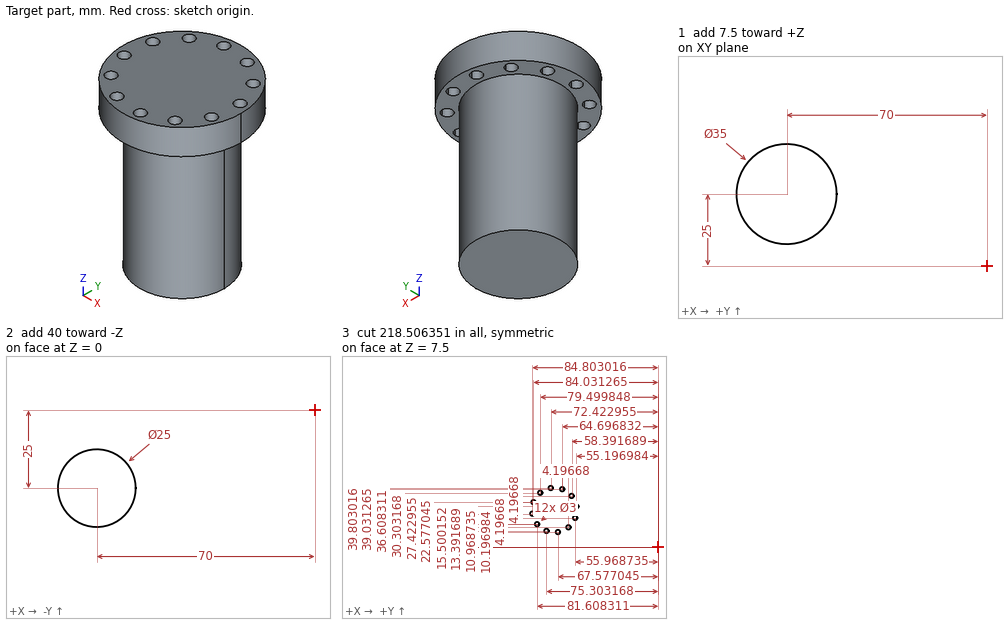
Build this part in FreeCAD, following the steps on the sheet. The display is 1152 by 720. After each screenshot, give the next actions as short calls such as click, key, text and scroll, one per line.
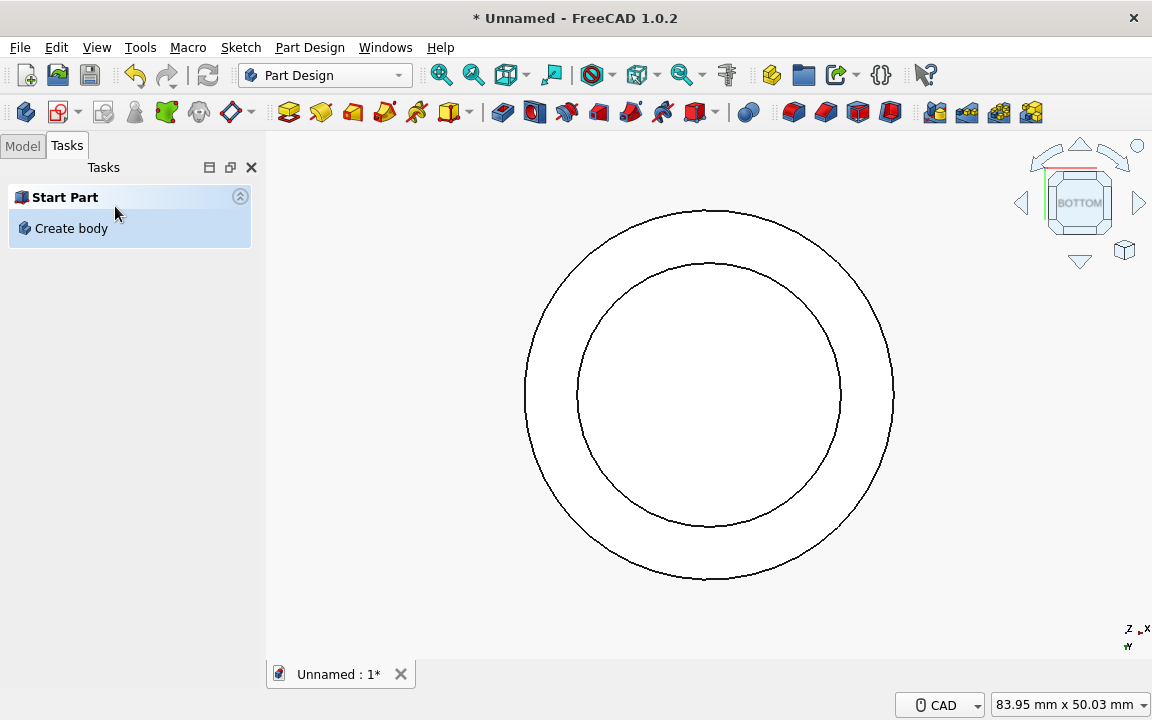
key(0)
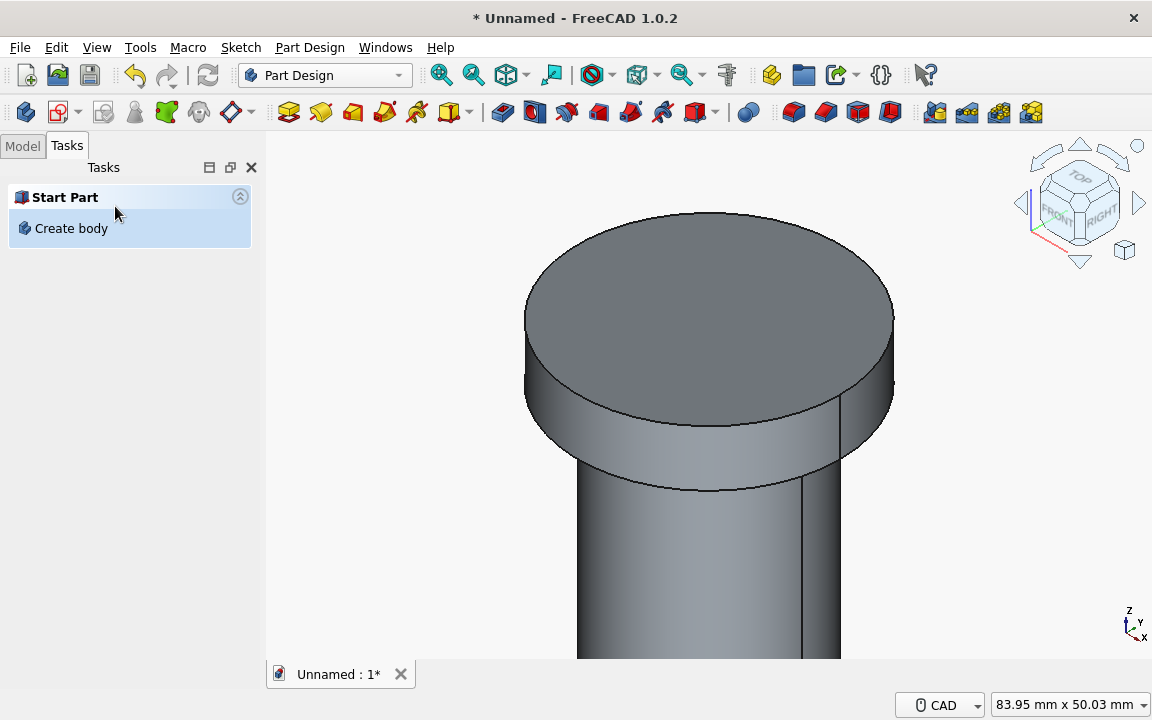
click(442, 76)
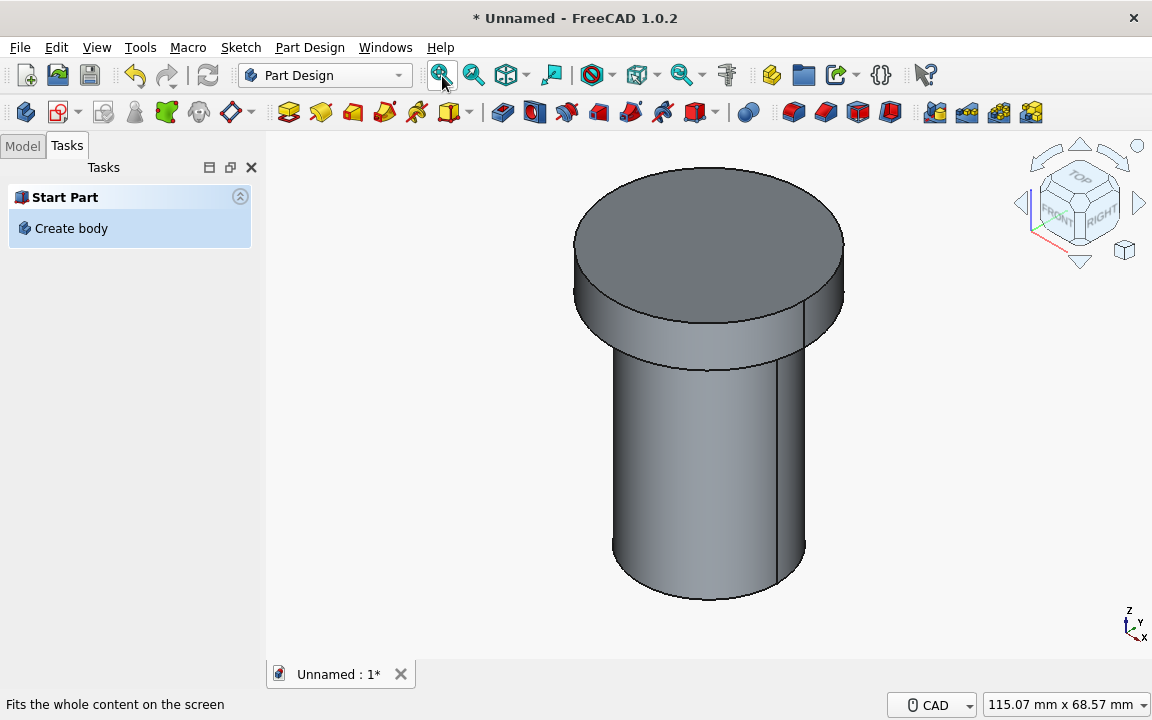
click(709, 245)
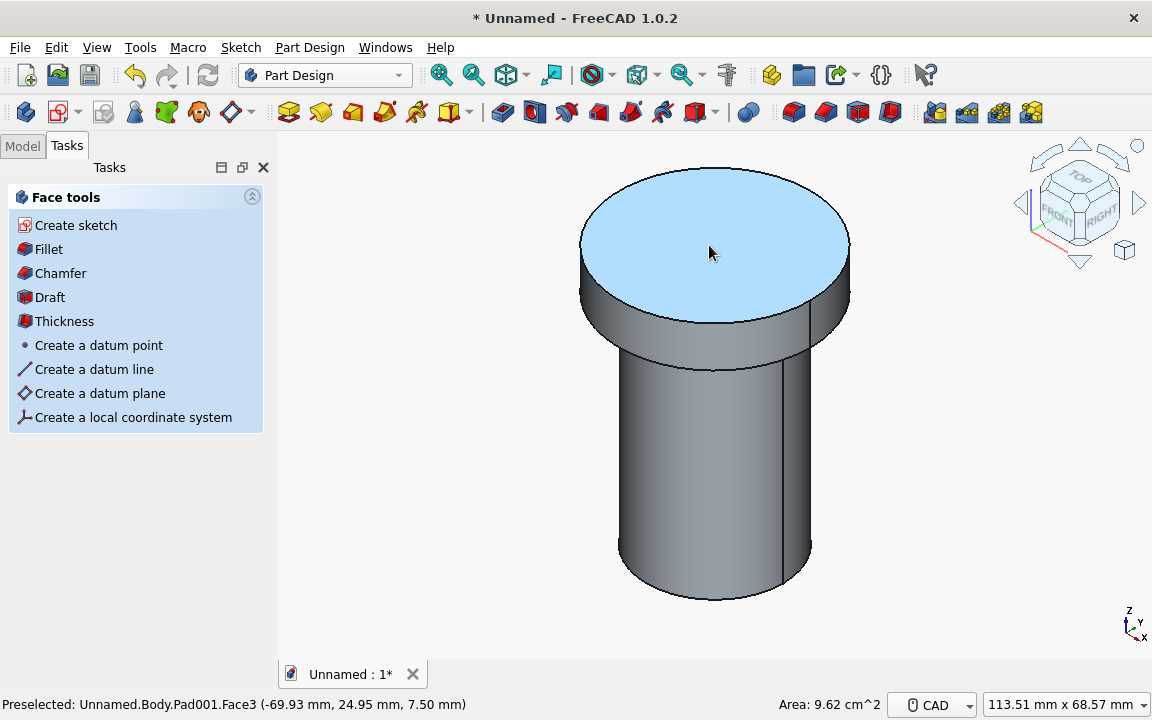
click(58, 112)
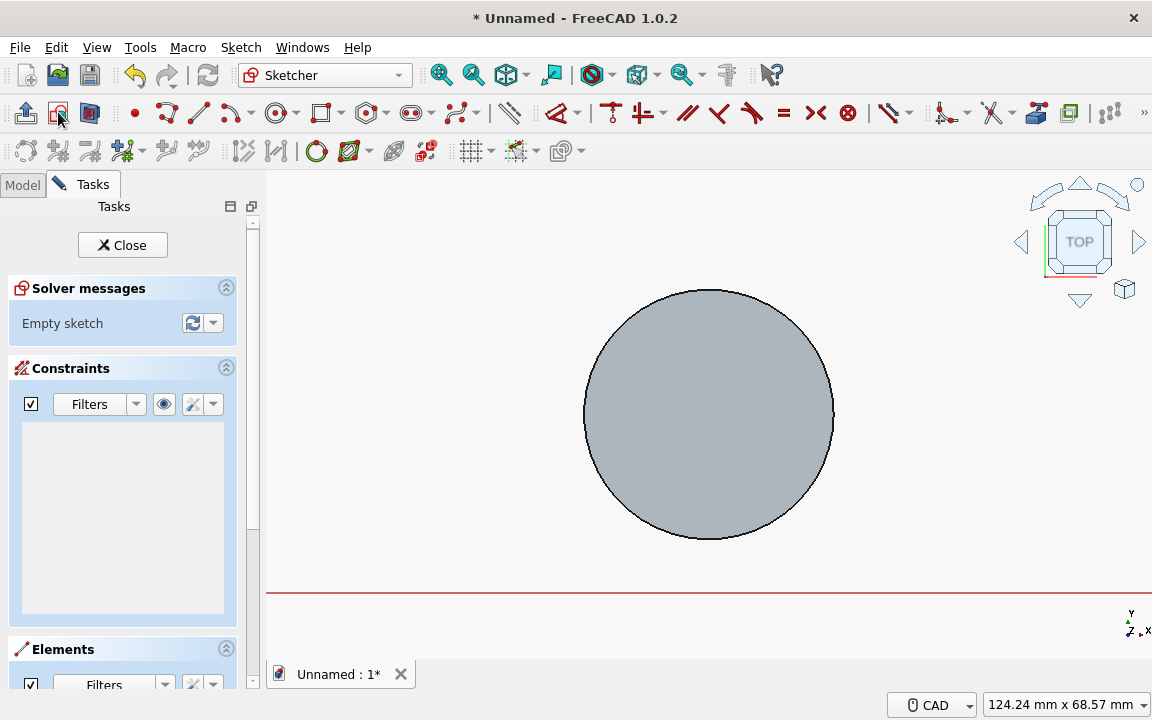
key(g)
key(c)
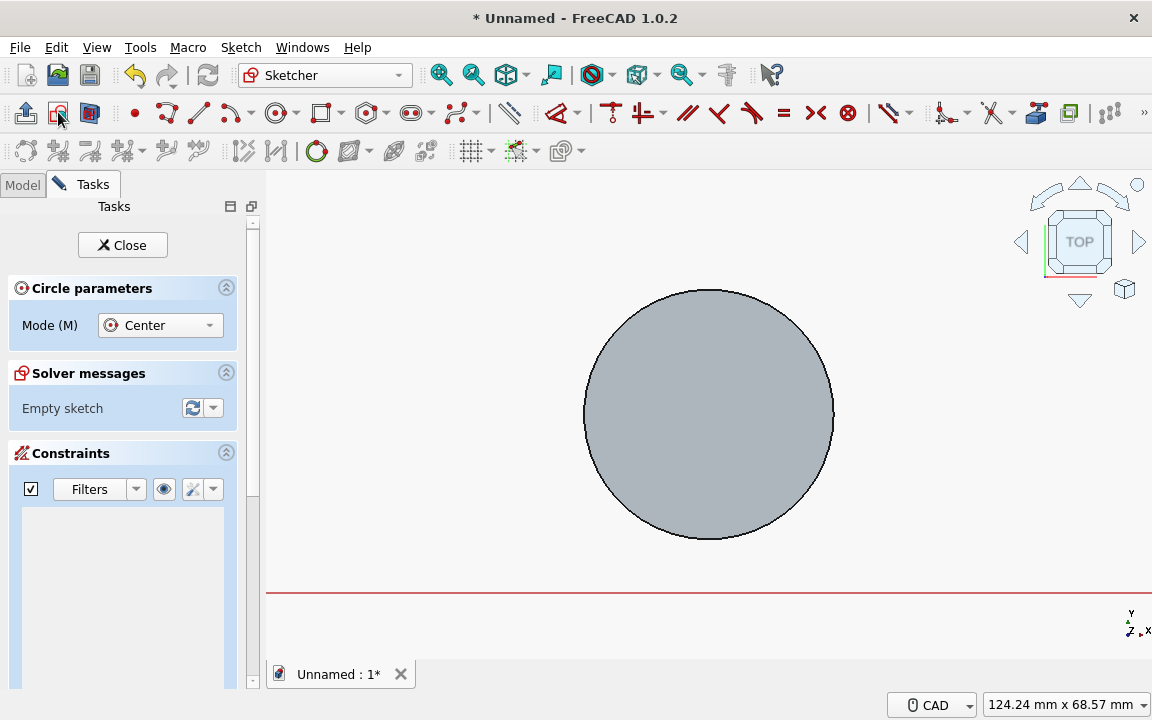
scroll(626, 482, up, 4)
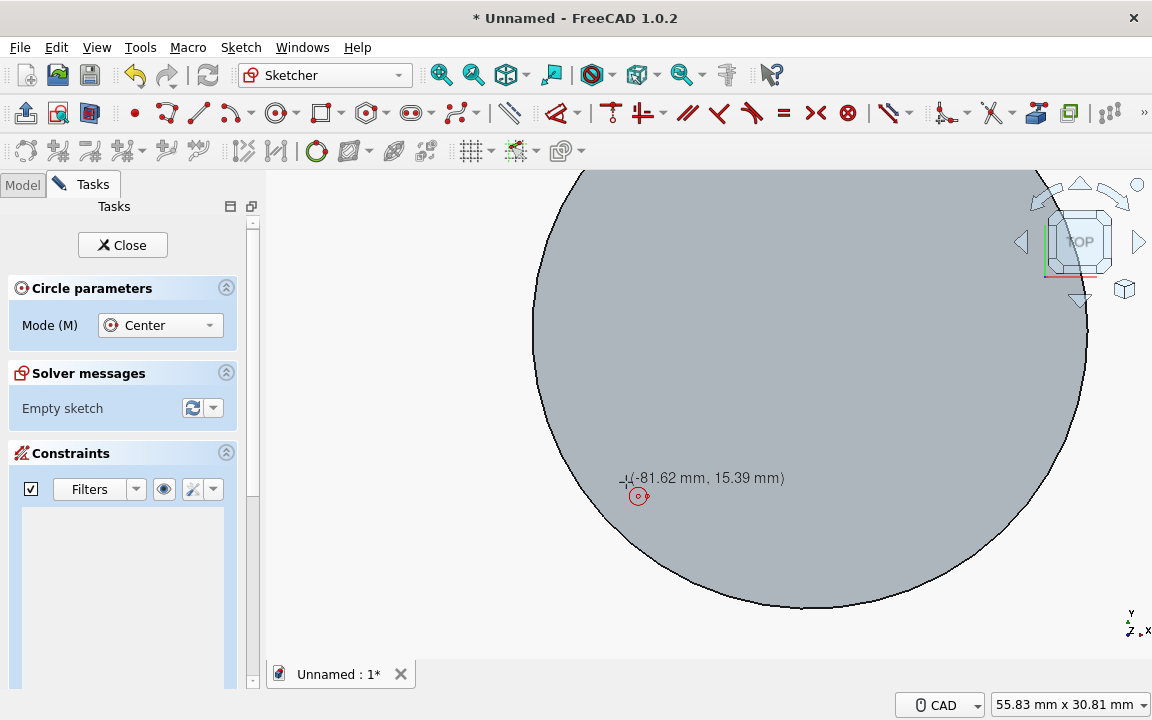
click(626, 482)
click(643, 465)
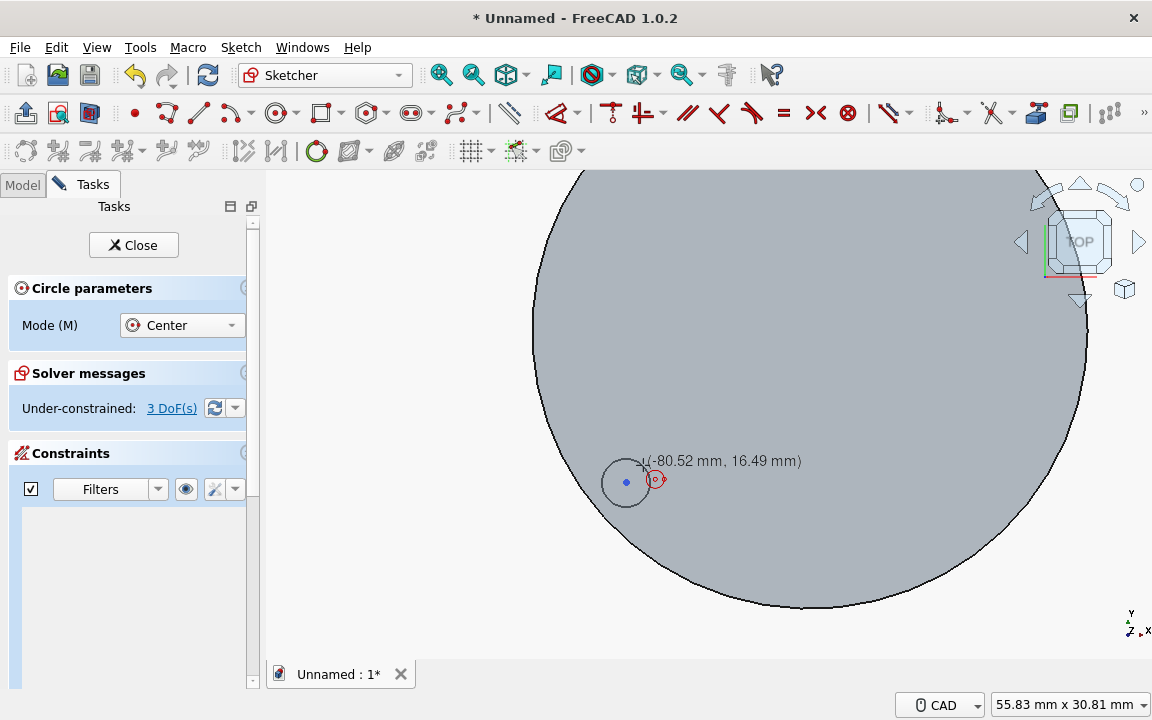
click(575, 369)
click(592, 353)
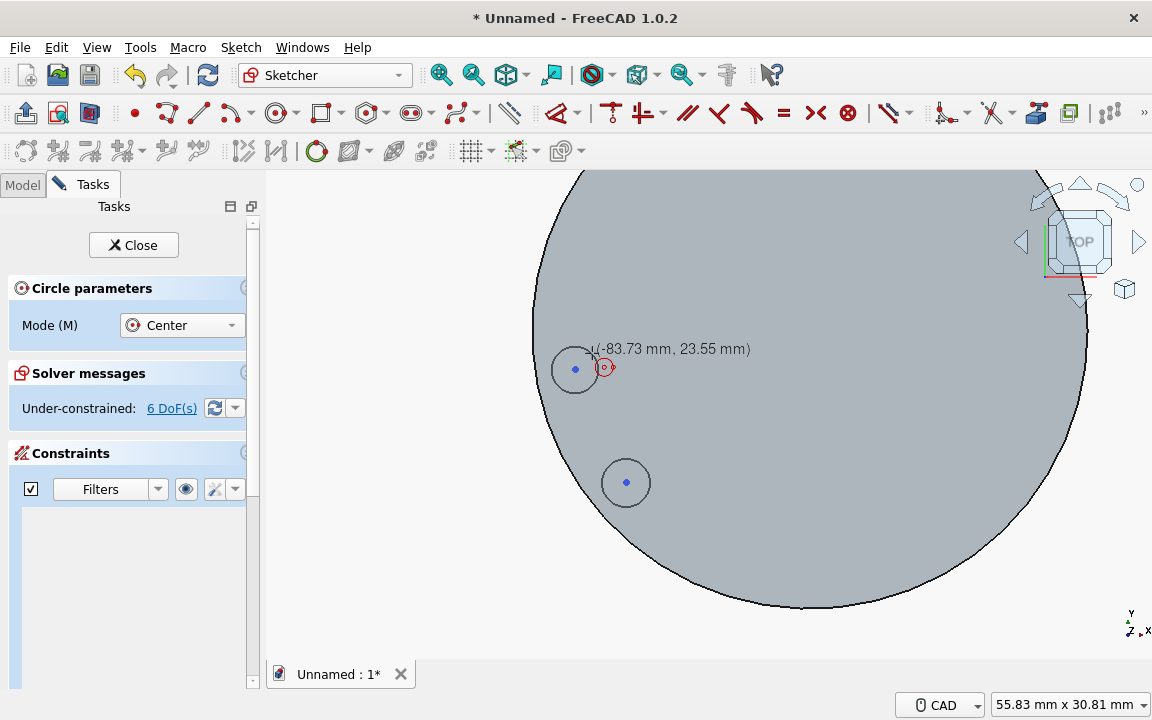
click(587, 247)
click(604, 230)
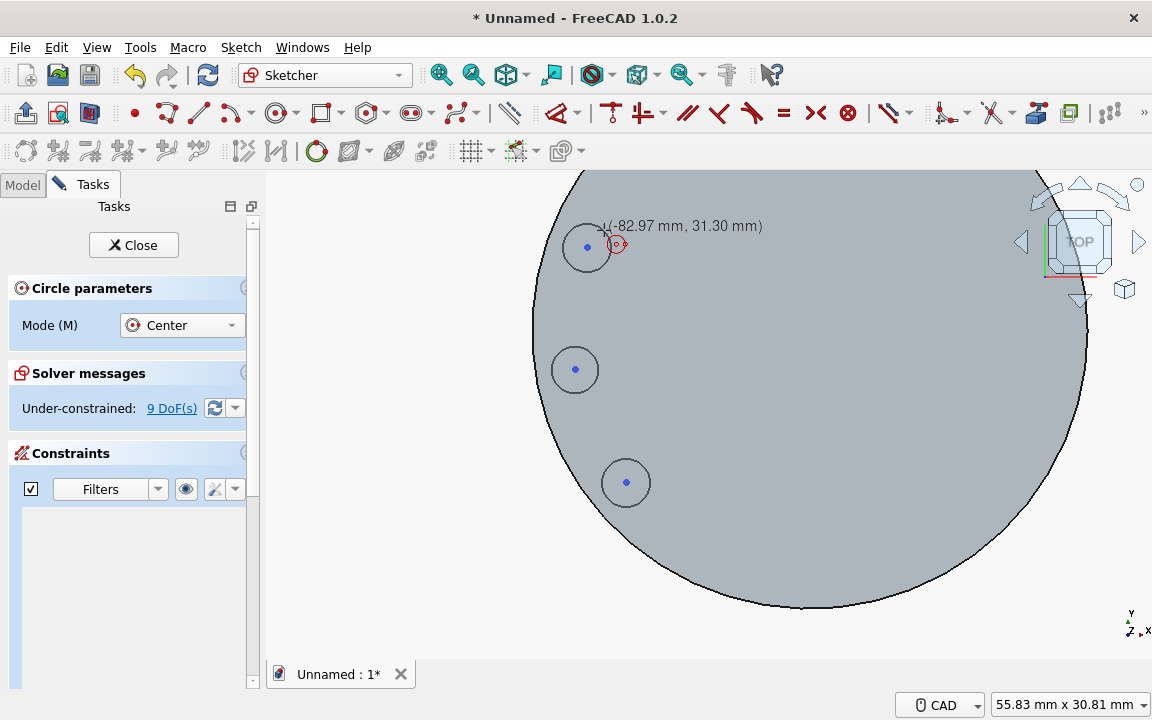
scroll(434, 516, down, 3)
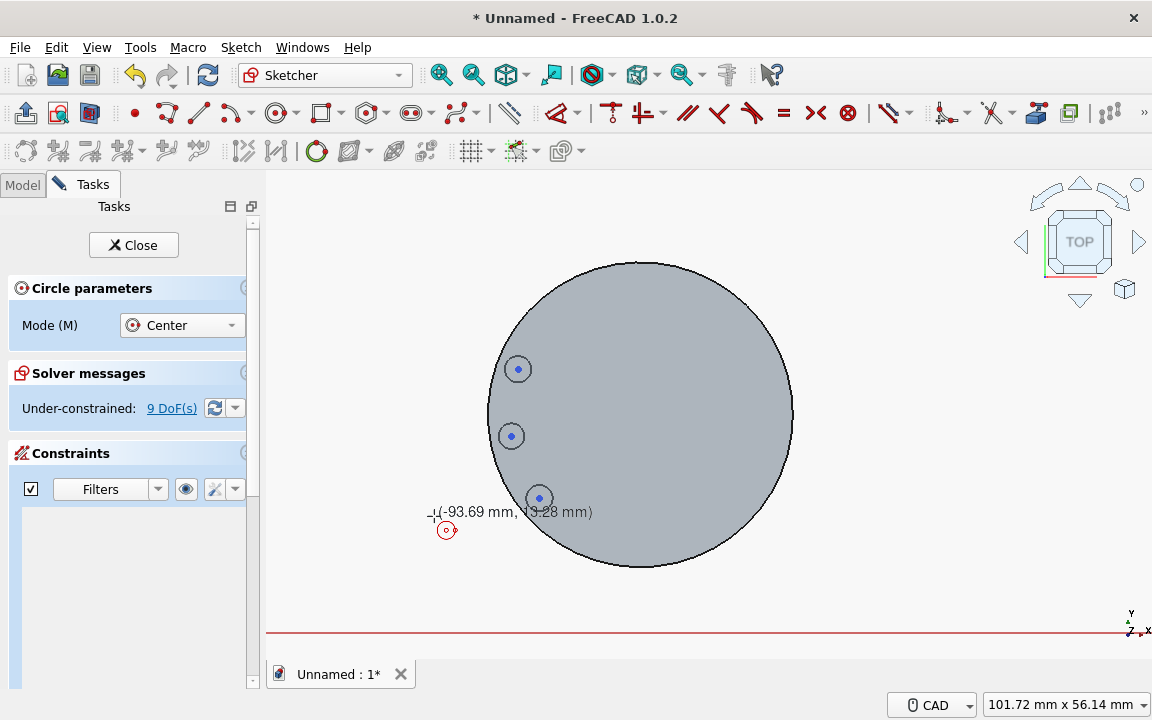
scroll(558, 314, up, 3)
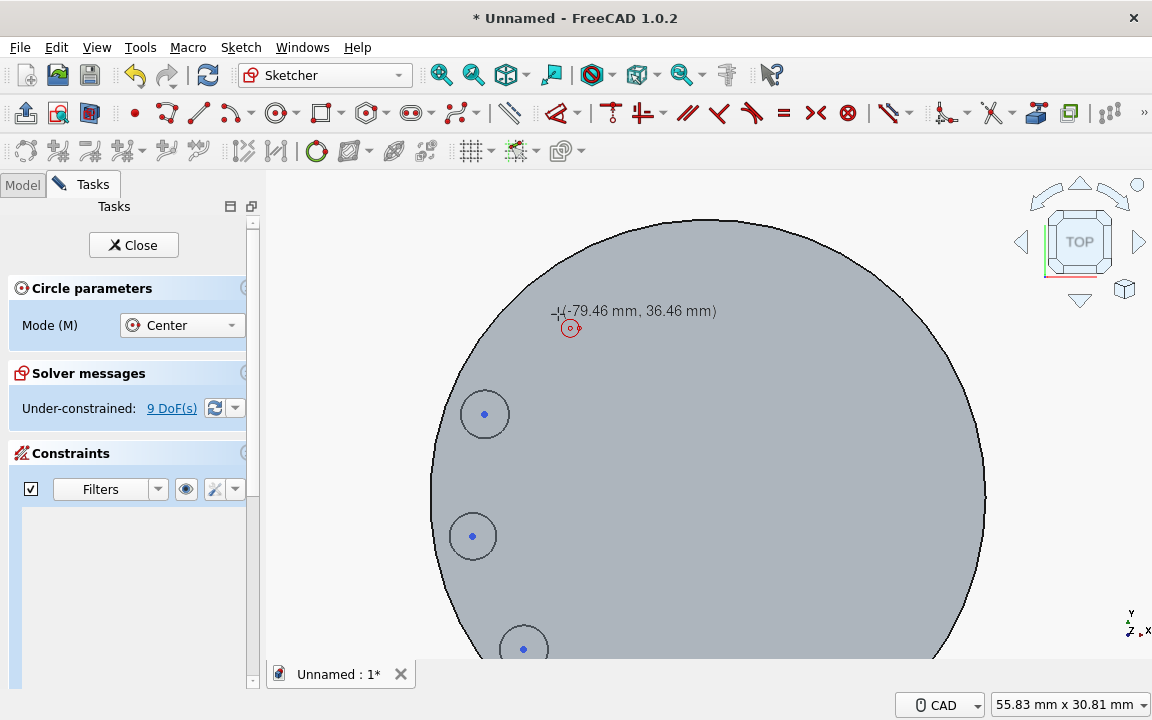
click(557, 313)
click(574, 296)